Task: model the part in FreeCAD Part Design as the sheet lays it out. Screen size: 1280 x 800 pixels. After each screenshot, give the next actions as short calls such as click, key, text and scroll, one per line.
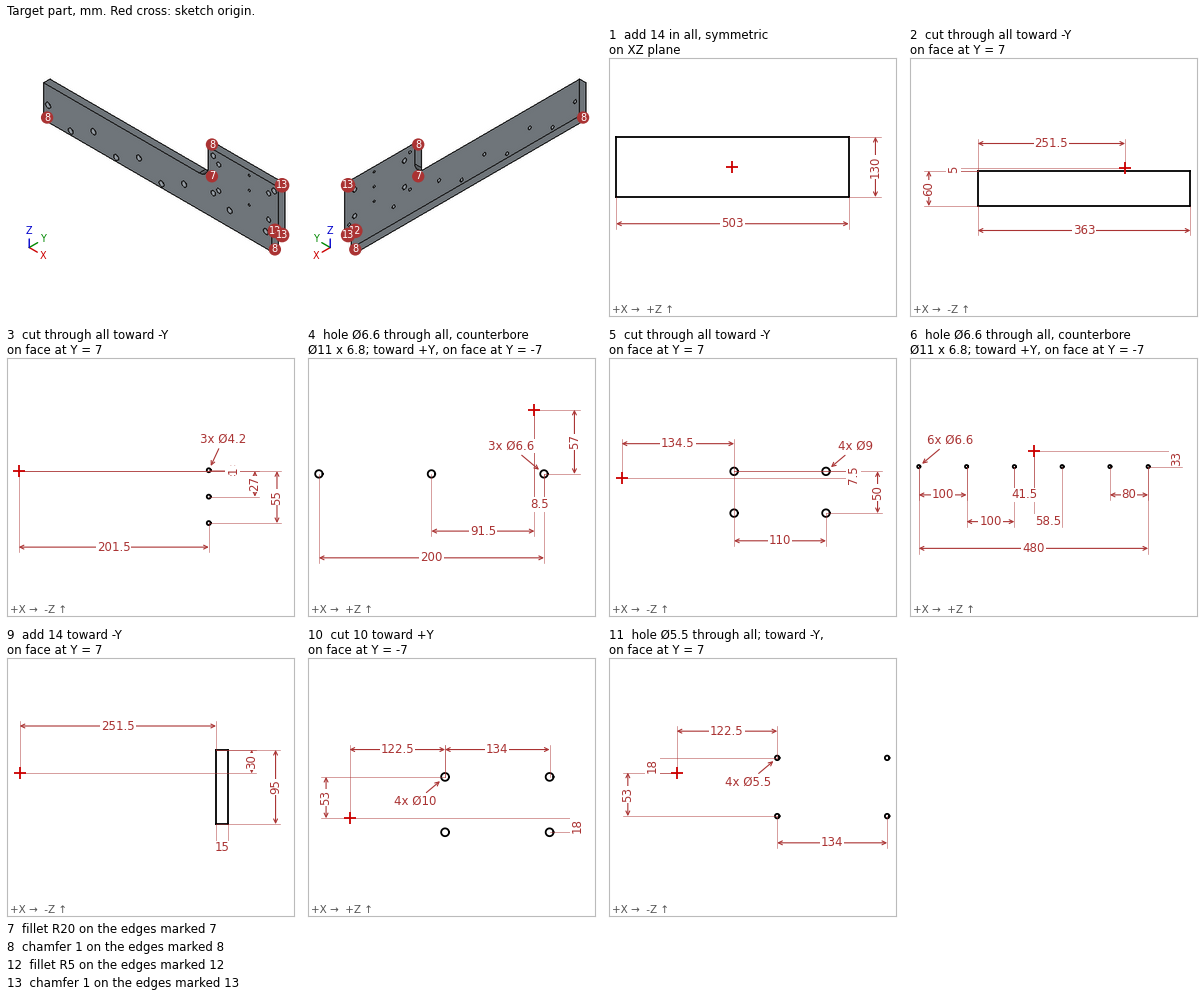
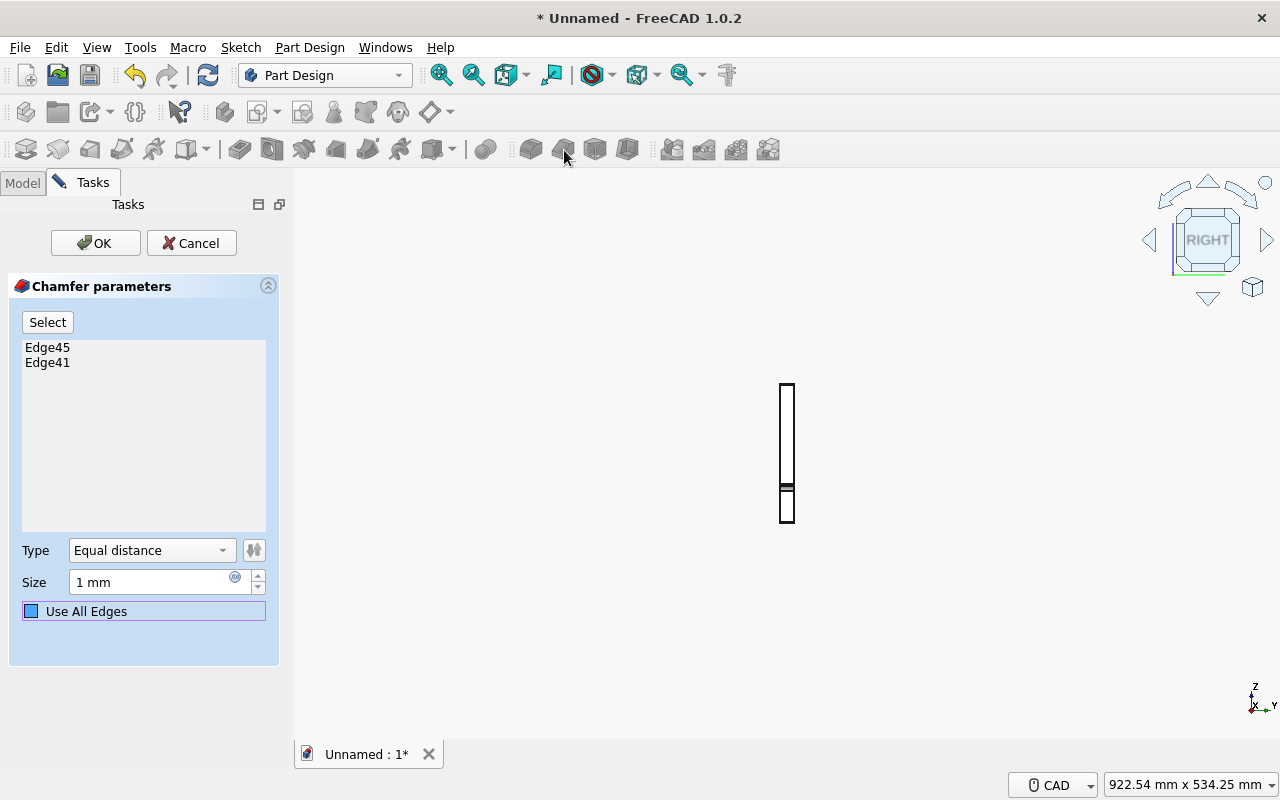
click(96, 243)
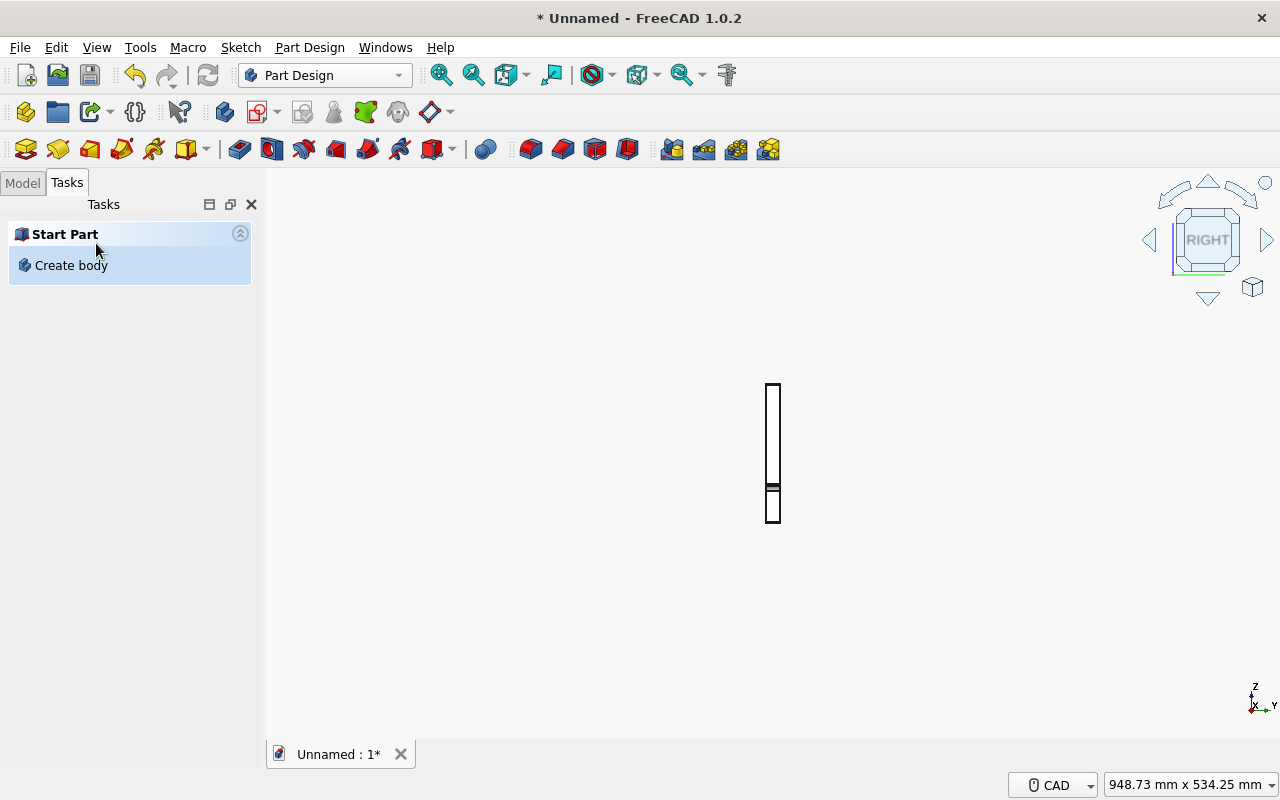
key(0)